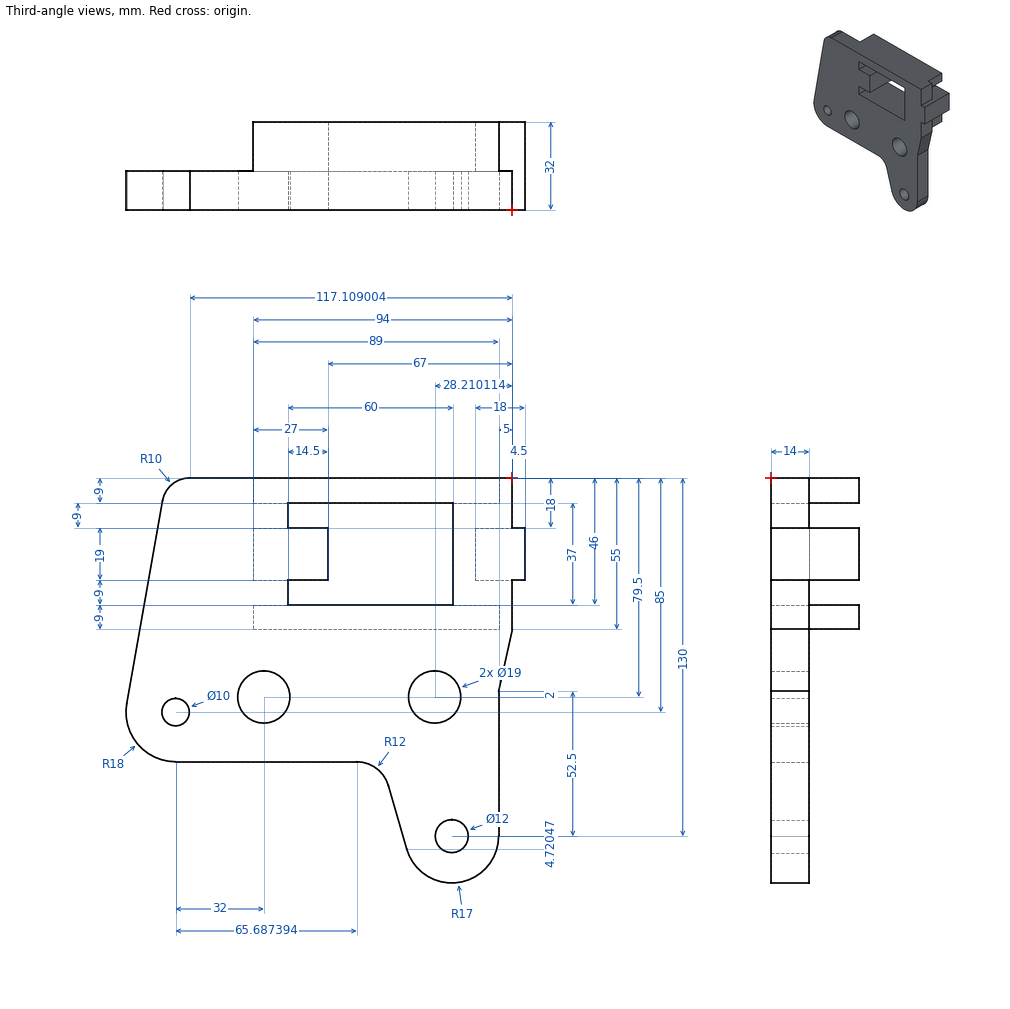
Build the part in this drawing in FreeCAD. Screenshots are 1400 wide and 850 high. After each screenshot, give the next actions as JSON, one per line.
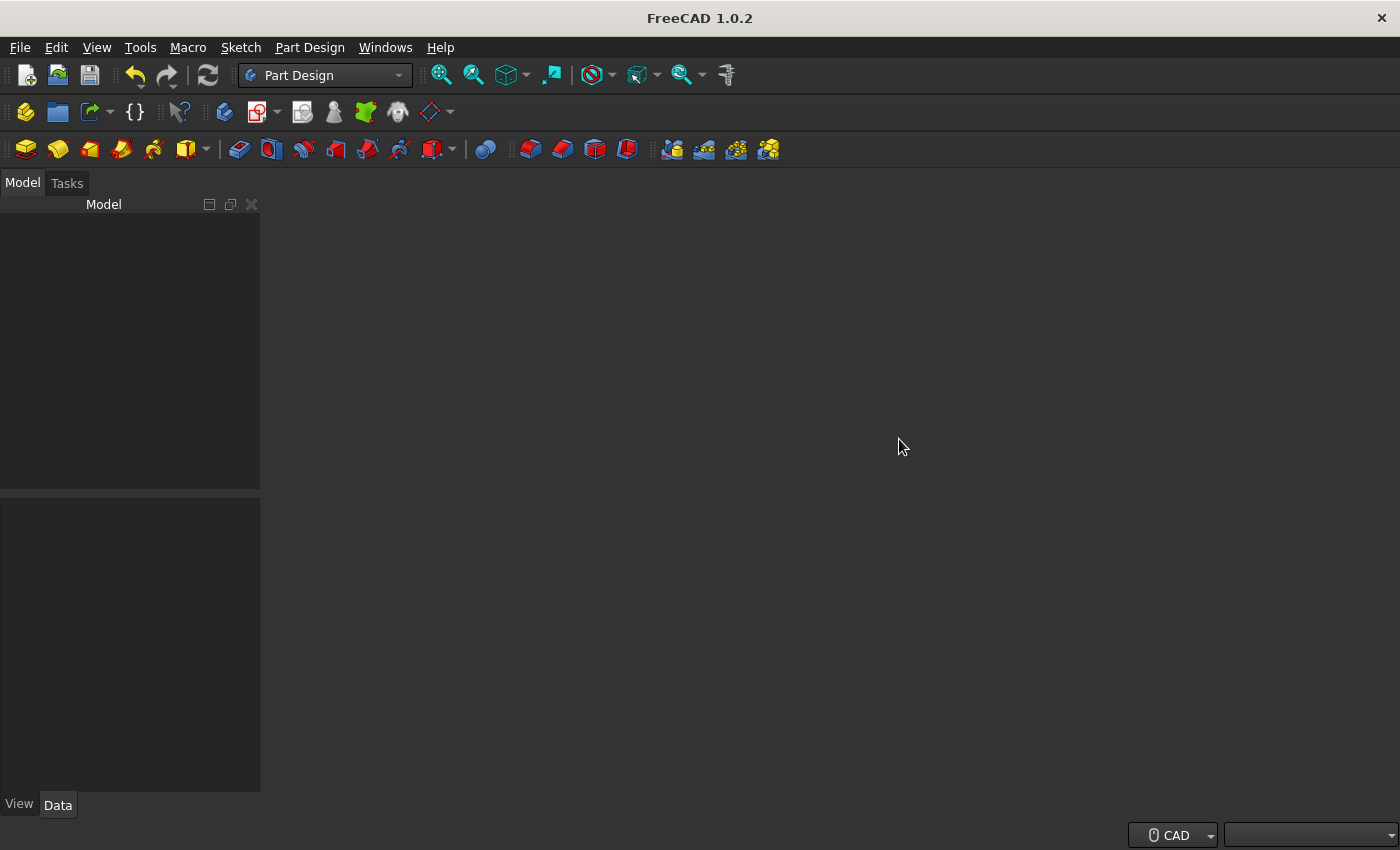
{"action": "left_click", "coordinate": [26, 76]}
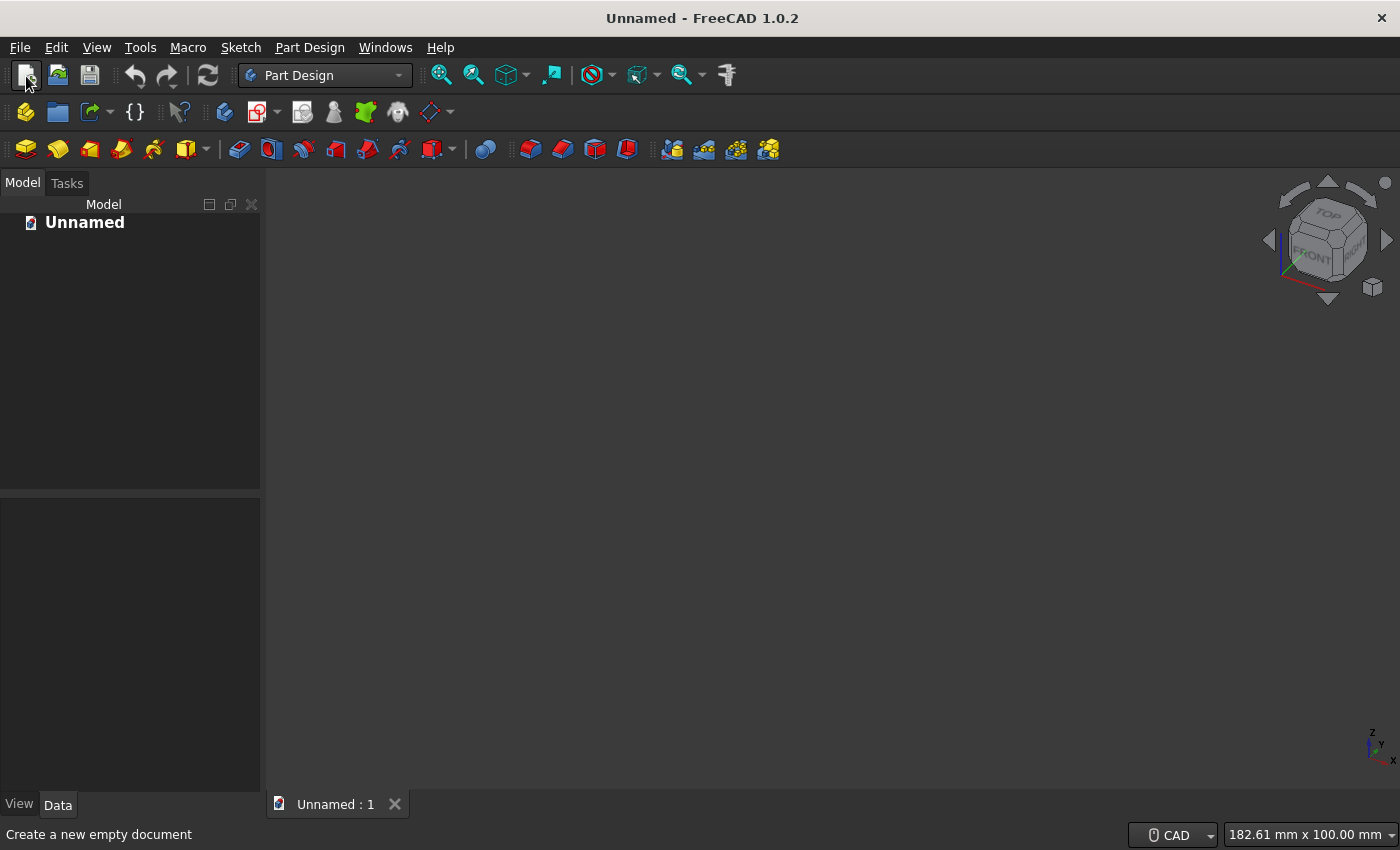
{"action": "left_click", "coordinate": [258, 112]}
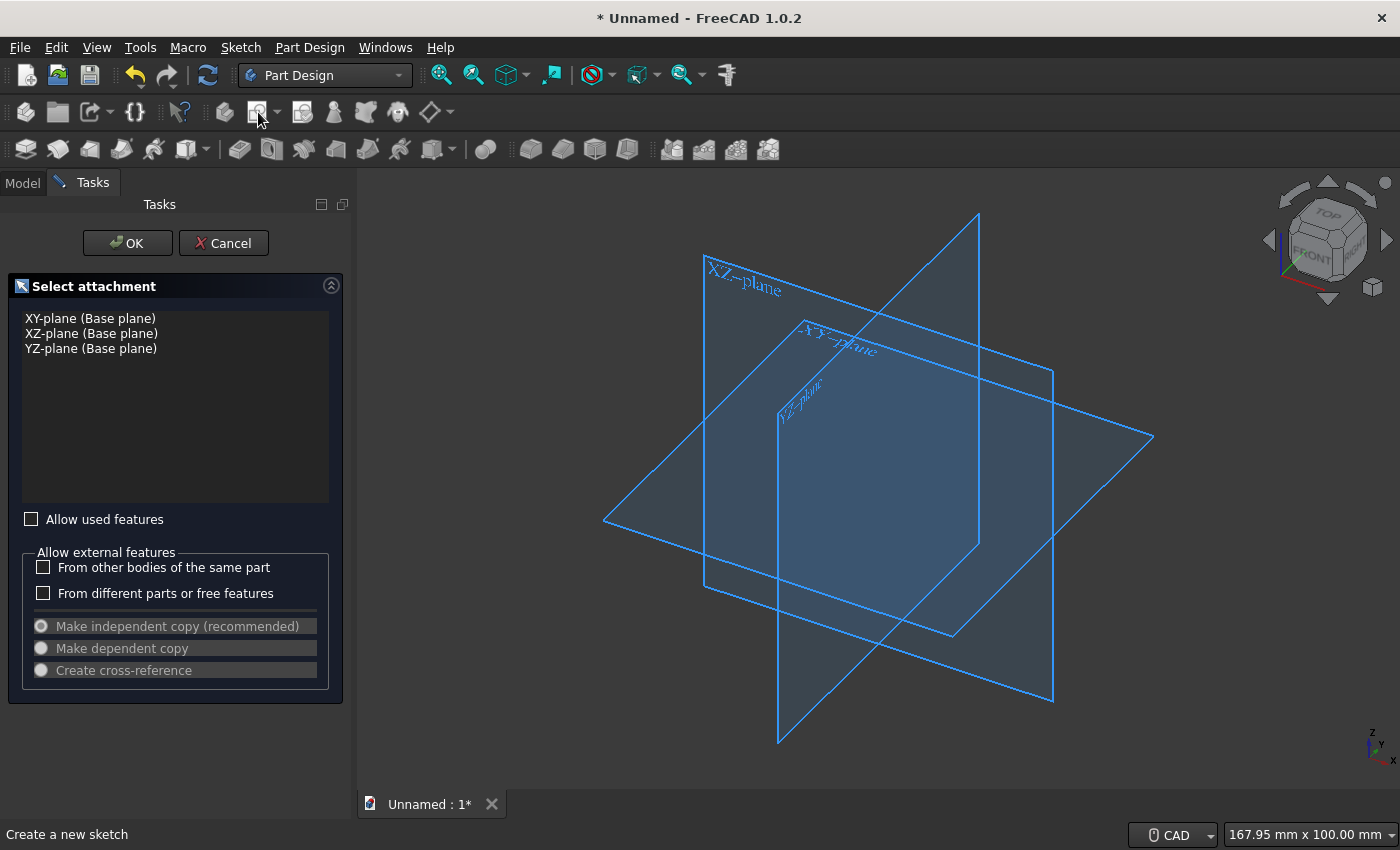
{"action": "left_click", "coordinate": [82, 334]}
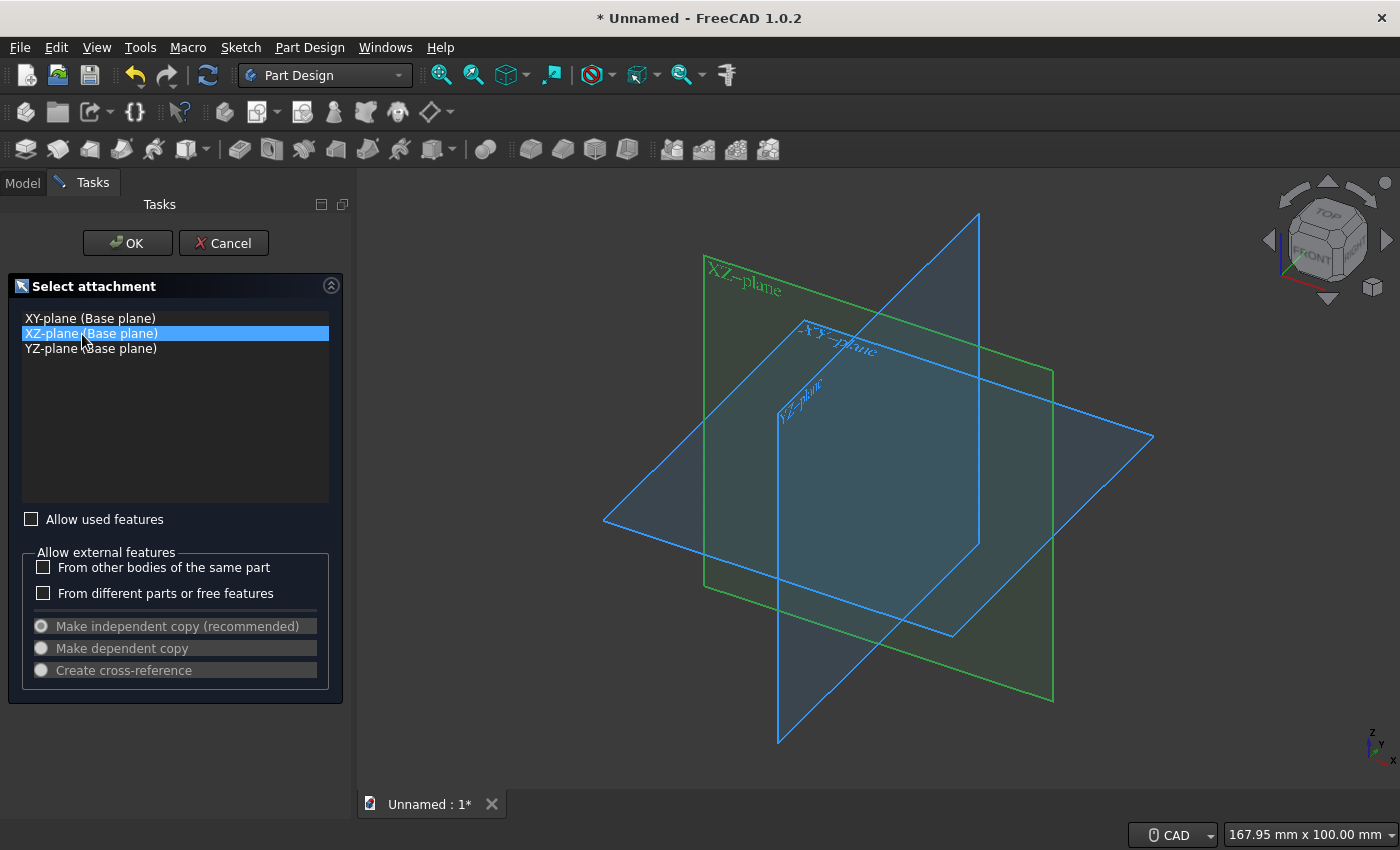
{"action": "left_click", "coordinate": [128, 243]}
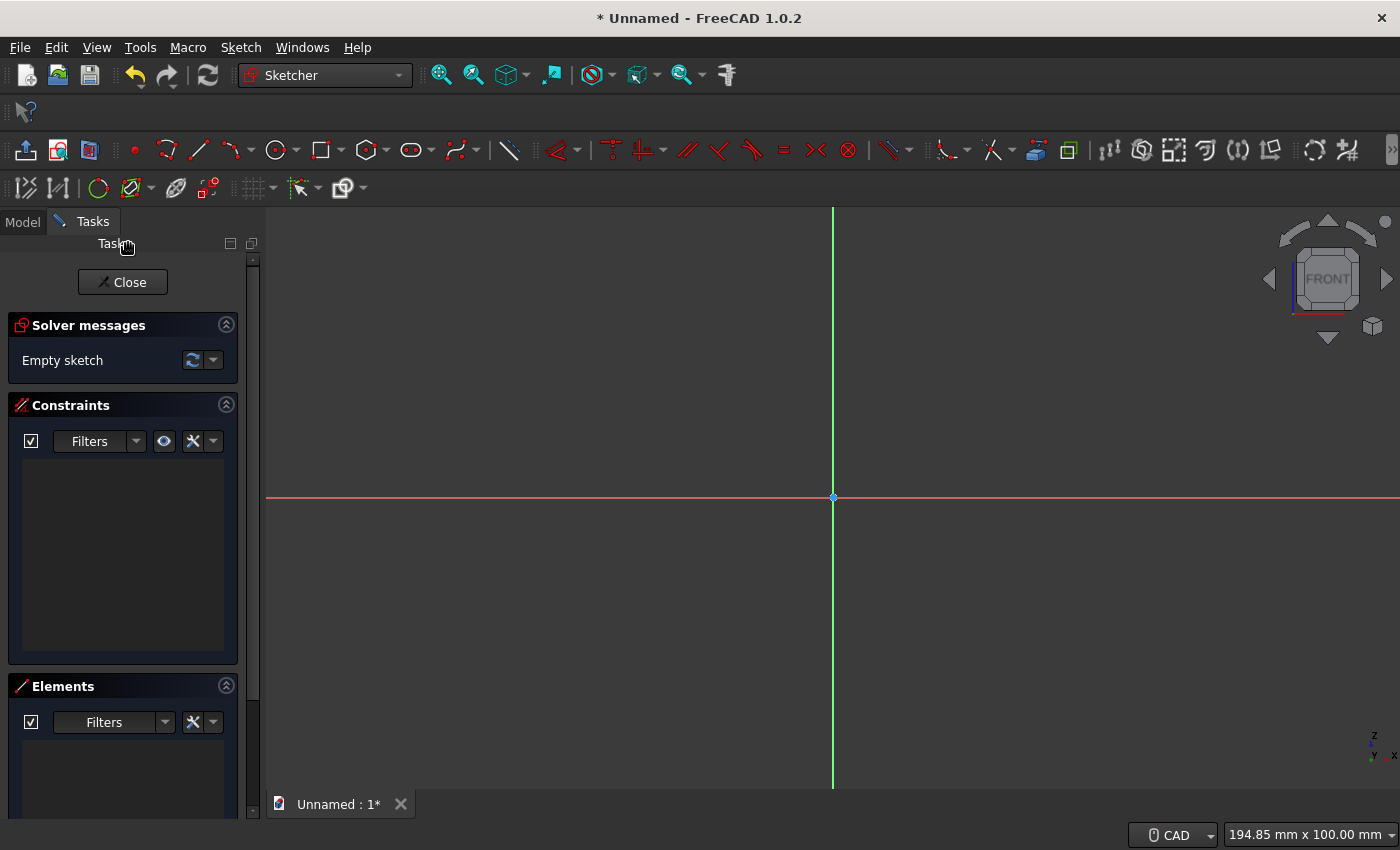
{"action": "scroll", "coordinate": [962, 249], "scroll_direction": "down", "scroll_amount": 5}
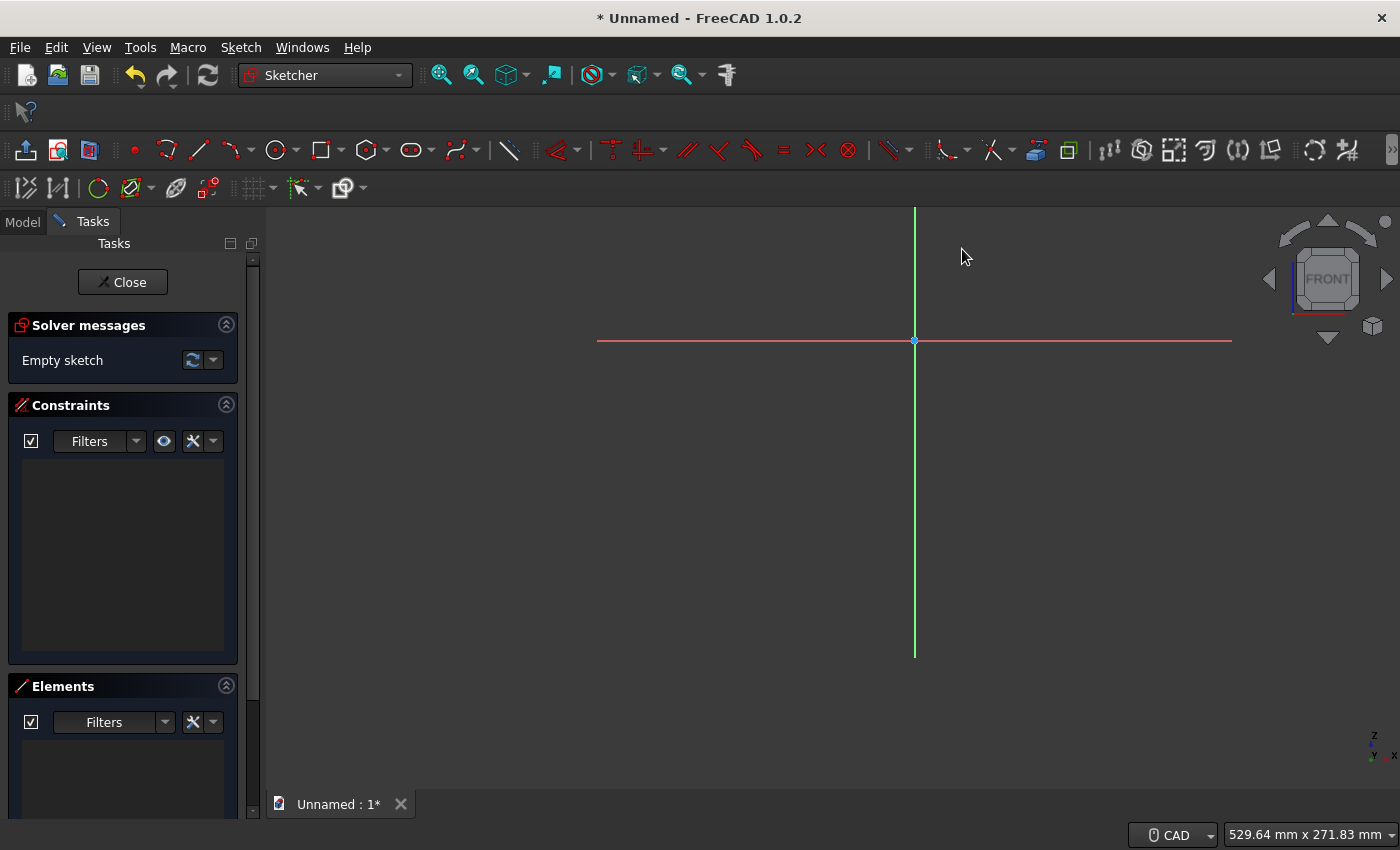
{"action": "left_click", "coordinate": [168, 150]}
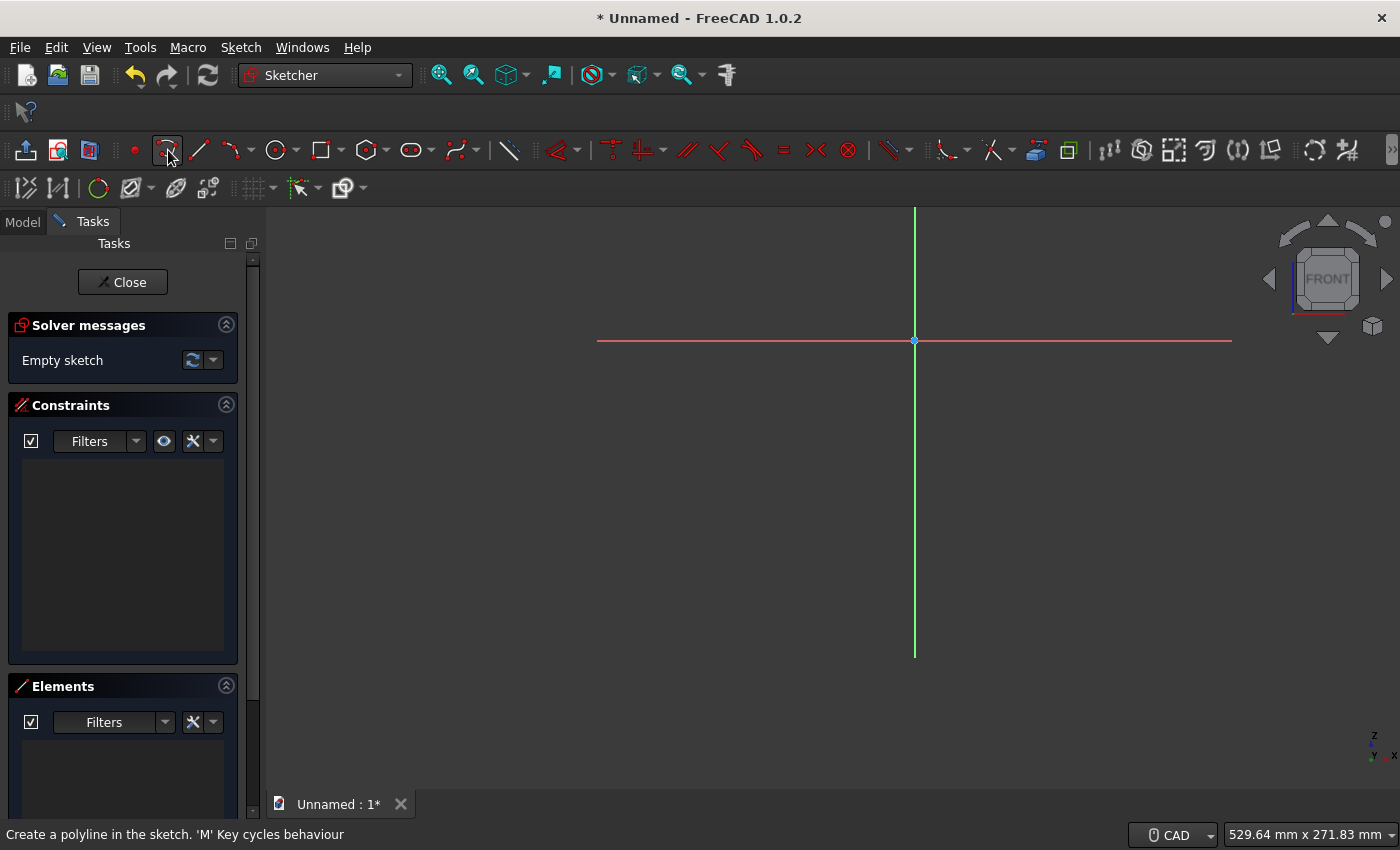
{"action": "left_click", "coordinate": [664, 341]}
{"action": "left_click", "coordinate": [915, 341]}
{"action": "left_click", "coordinate": [906, 458]}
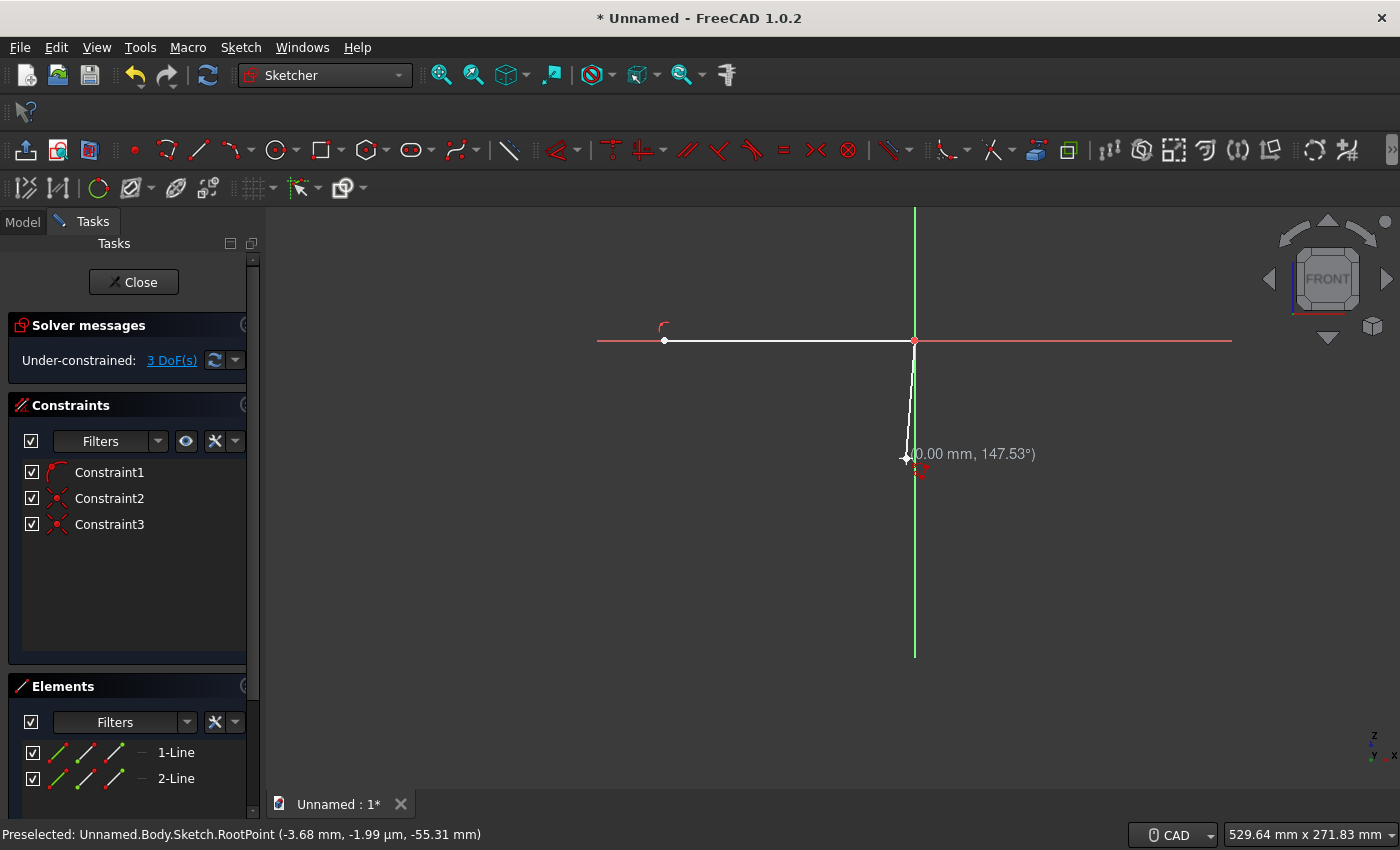
{"action": "scroll", "coordinate": [904, 507], "scroll_direction": "up", "scroll_amount": 2}